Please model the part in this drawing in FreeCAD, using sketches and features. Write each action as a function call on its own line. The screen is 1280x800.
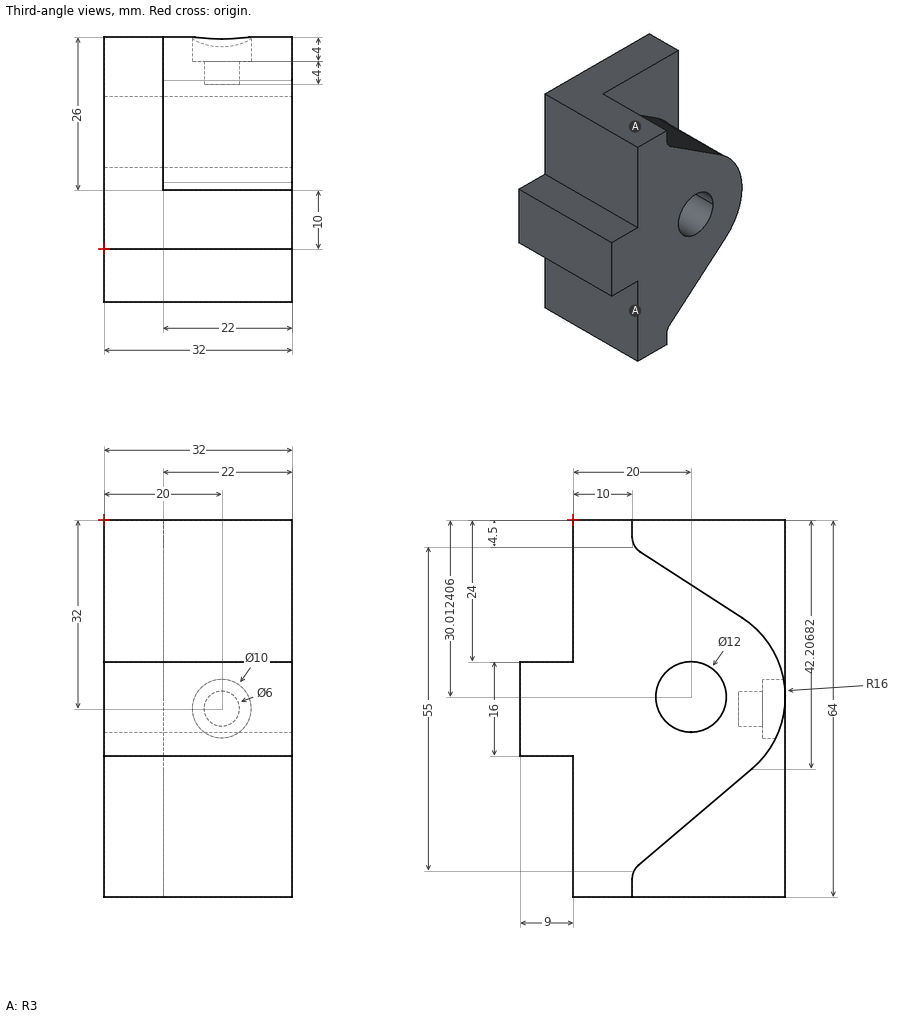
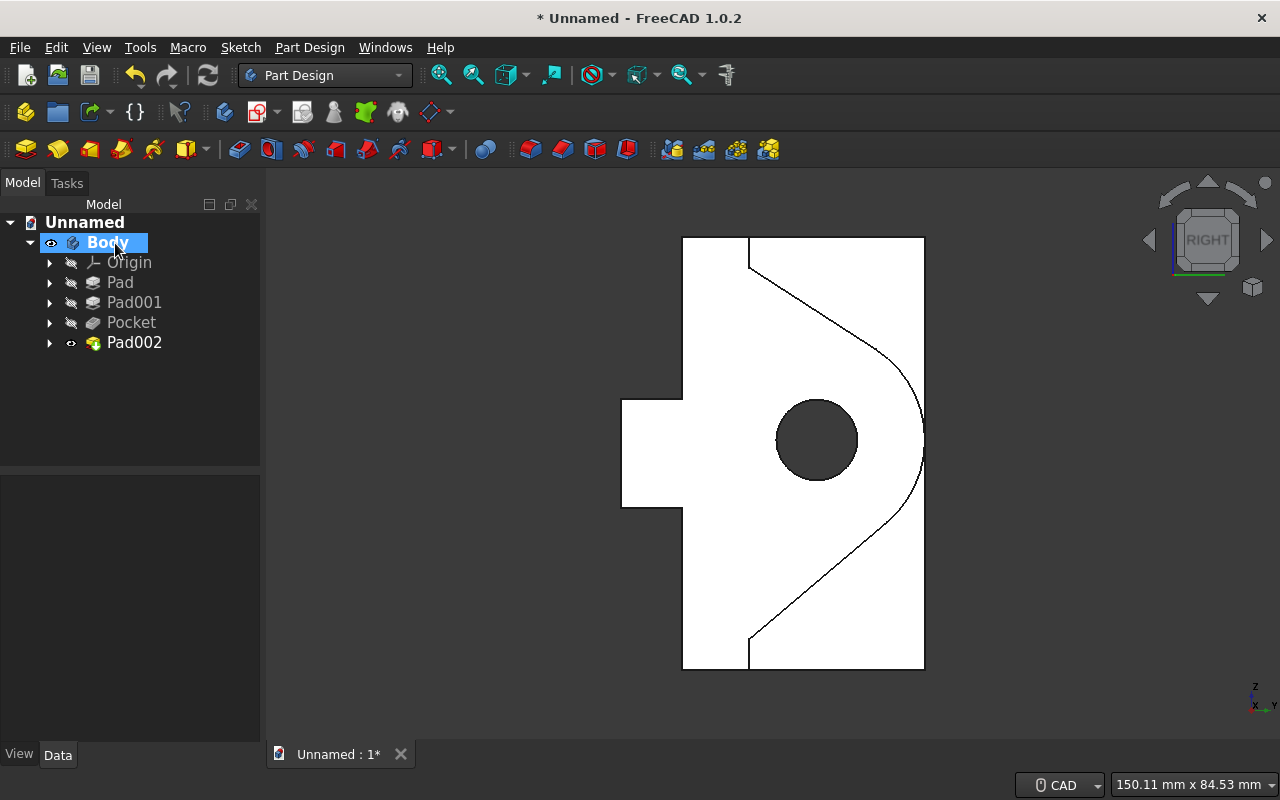
key(5)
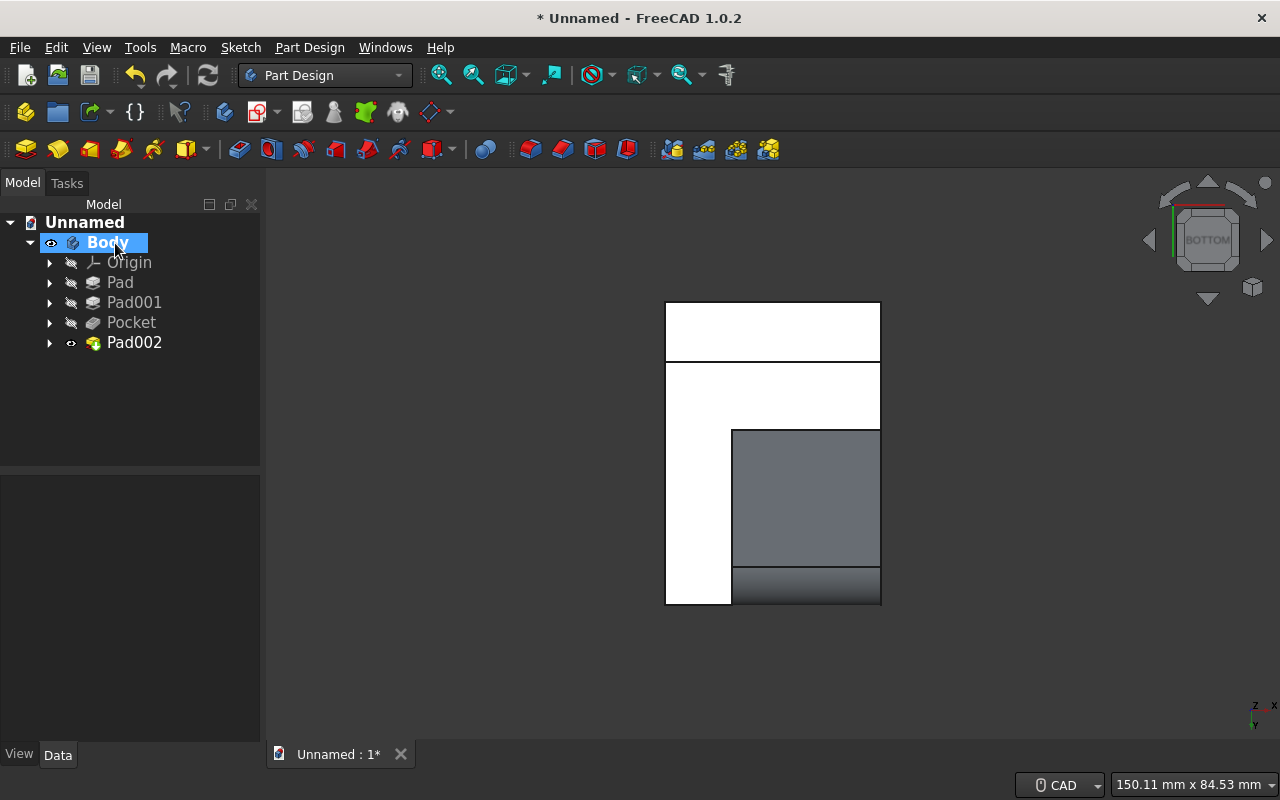
key(4)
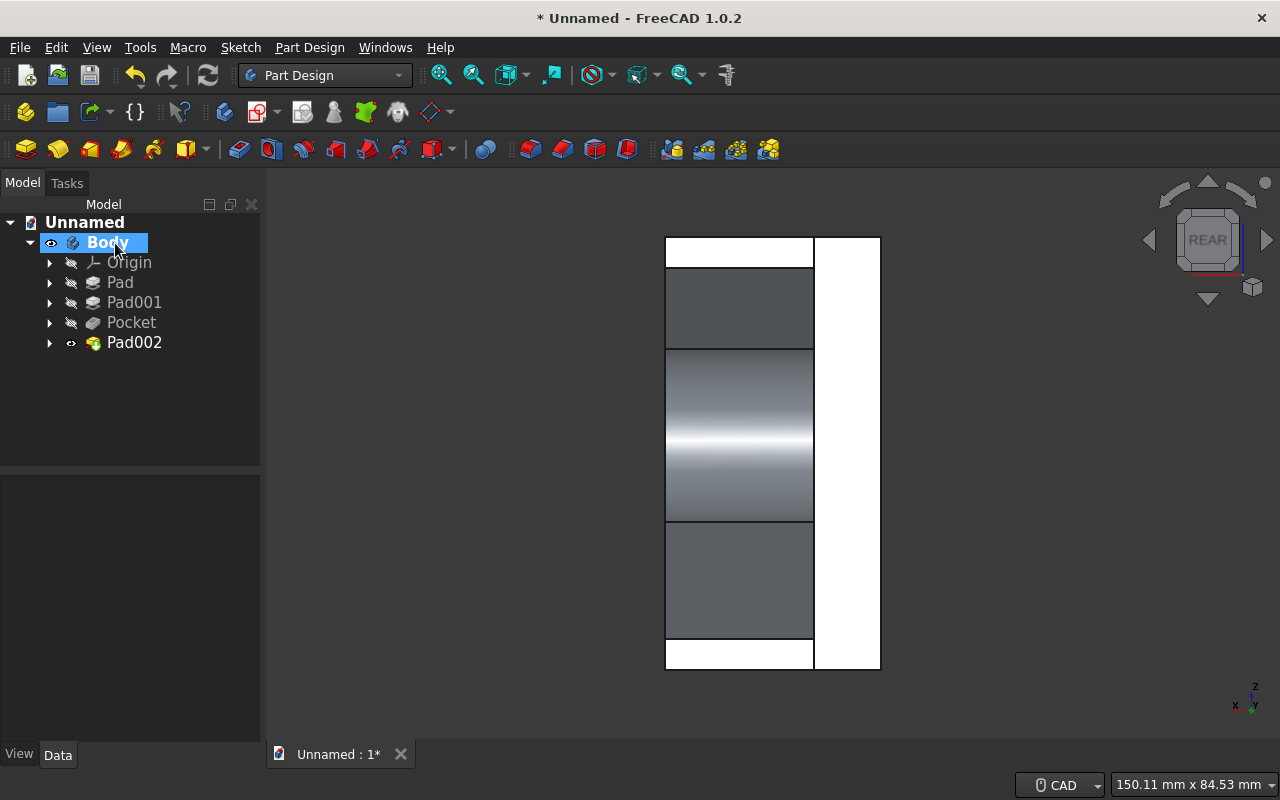
key(6)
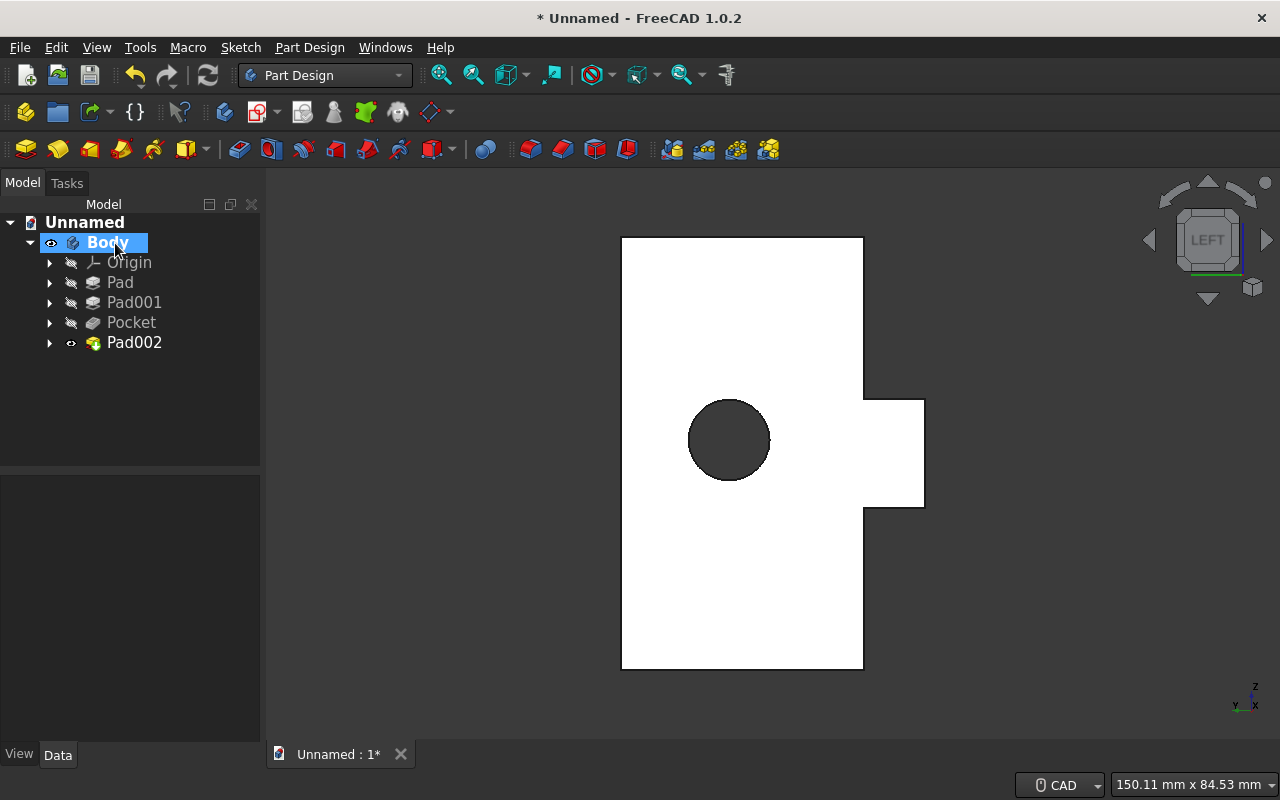
key(v)
key(3)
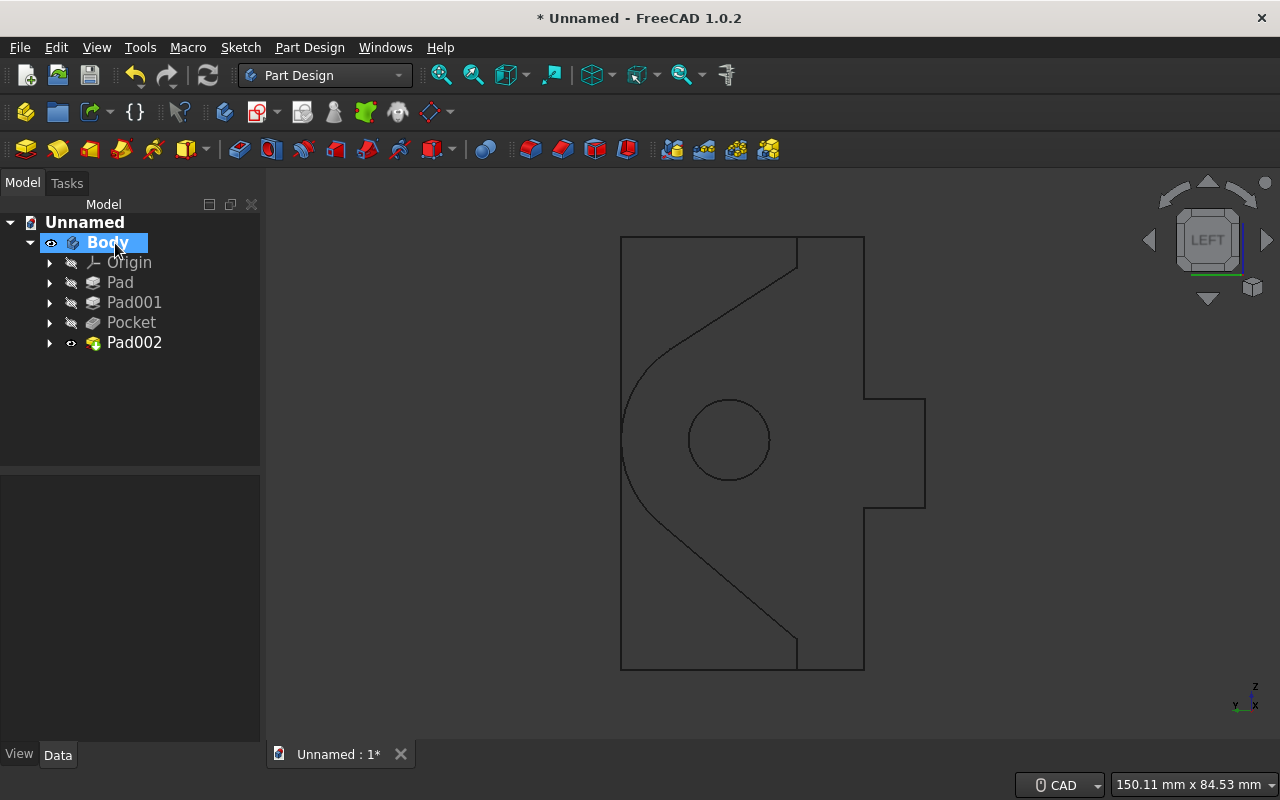
key(0)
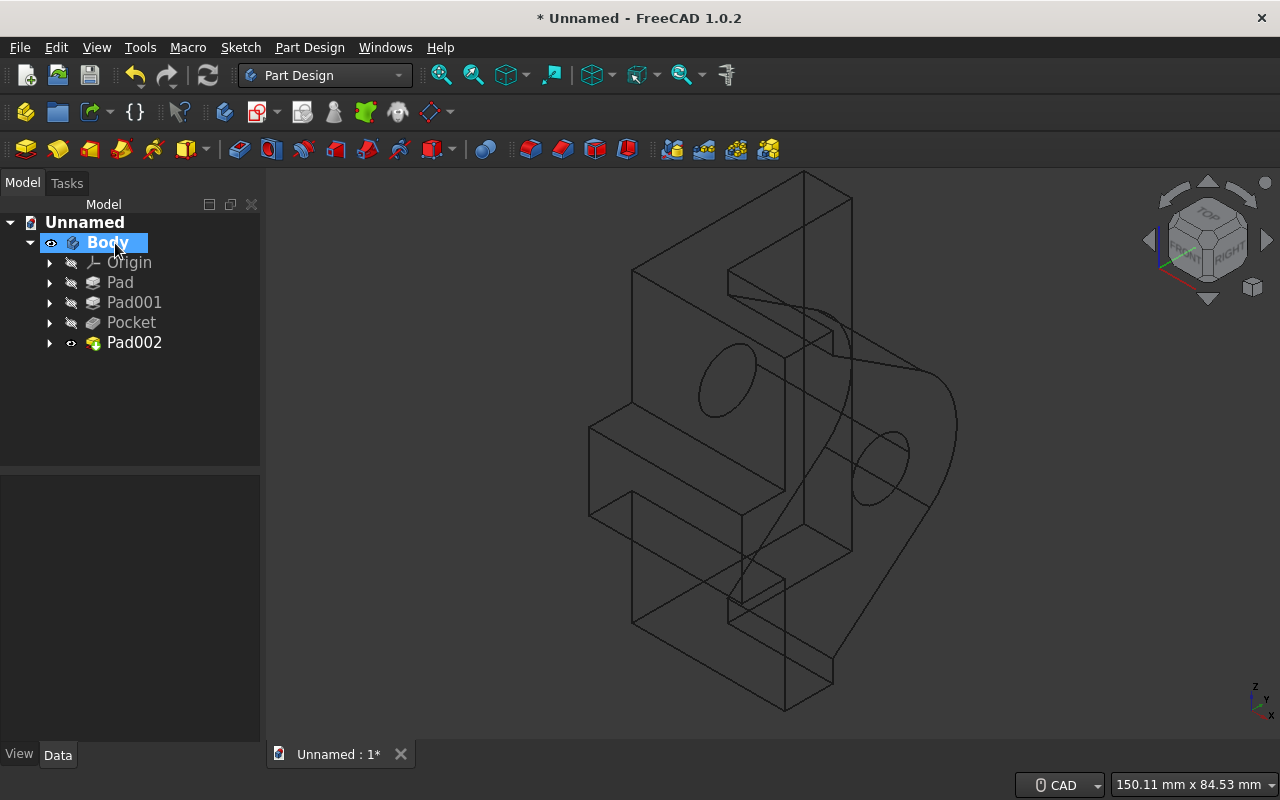
click(791, 634)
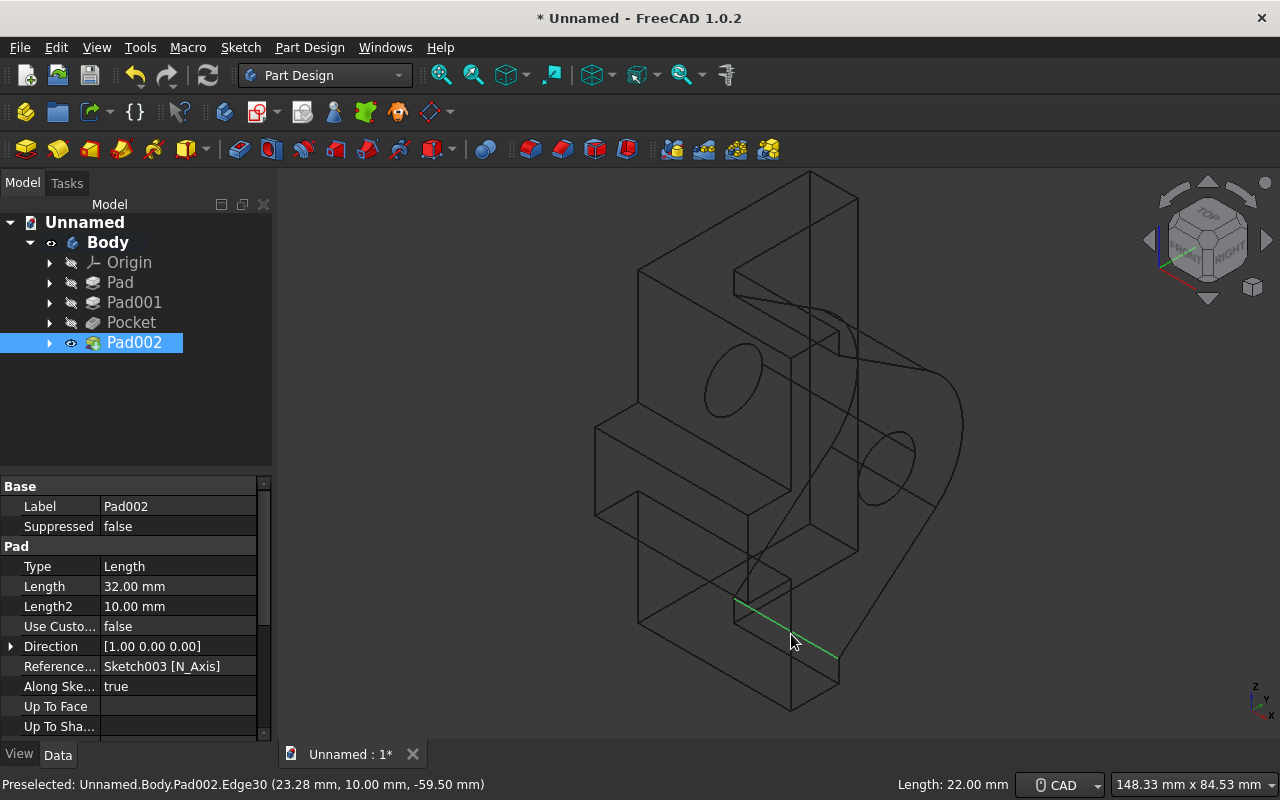
click(786, 324, ctrl)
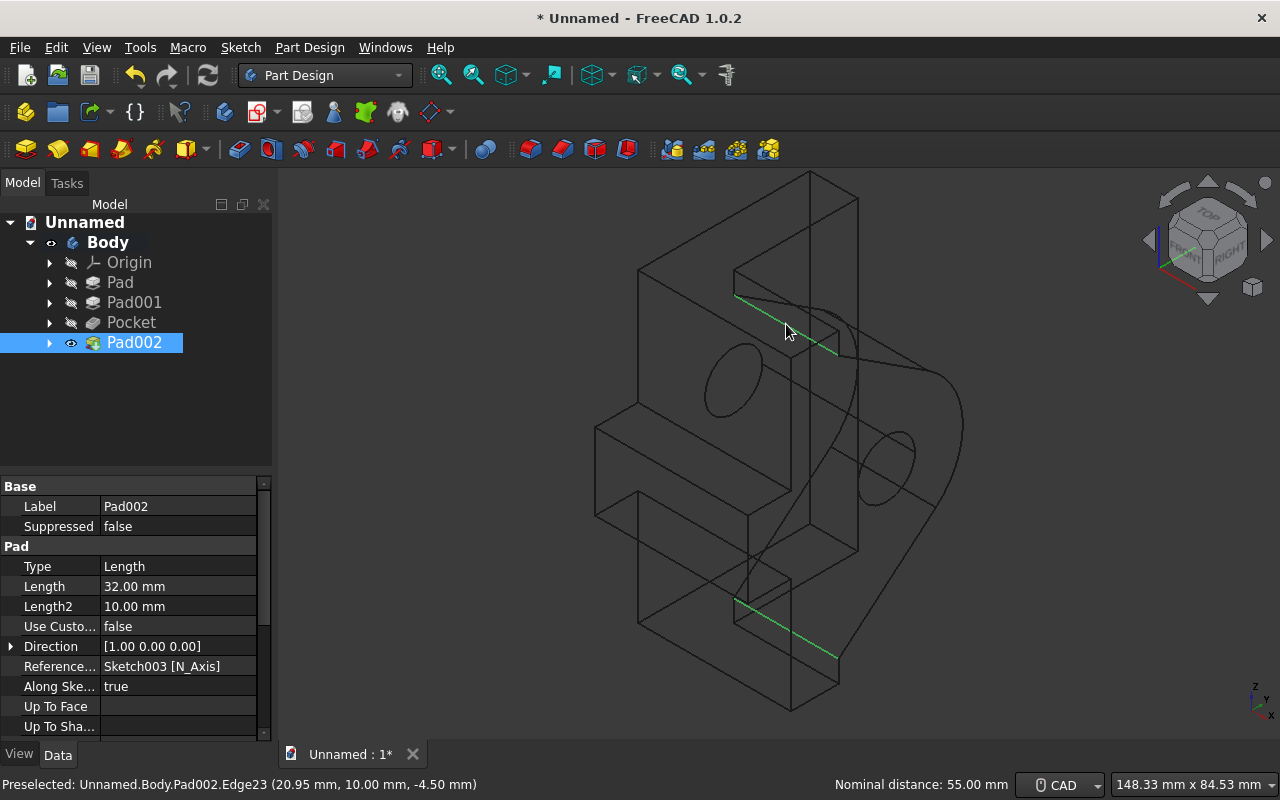
key(v)
key(1)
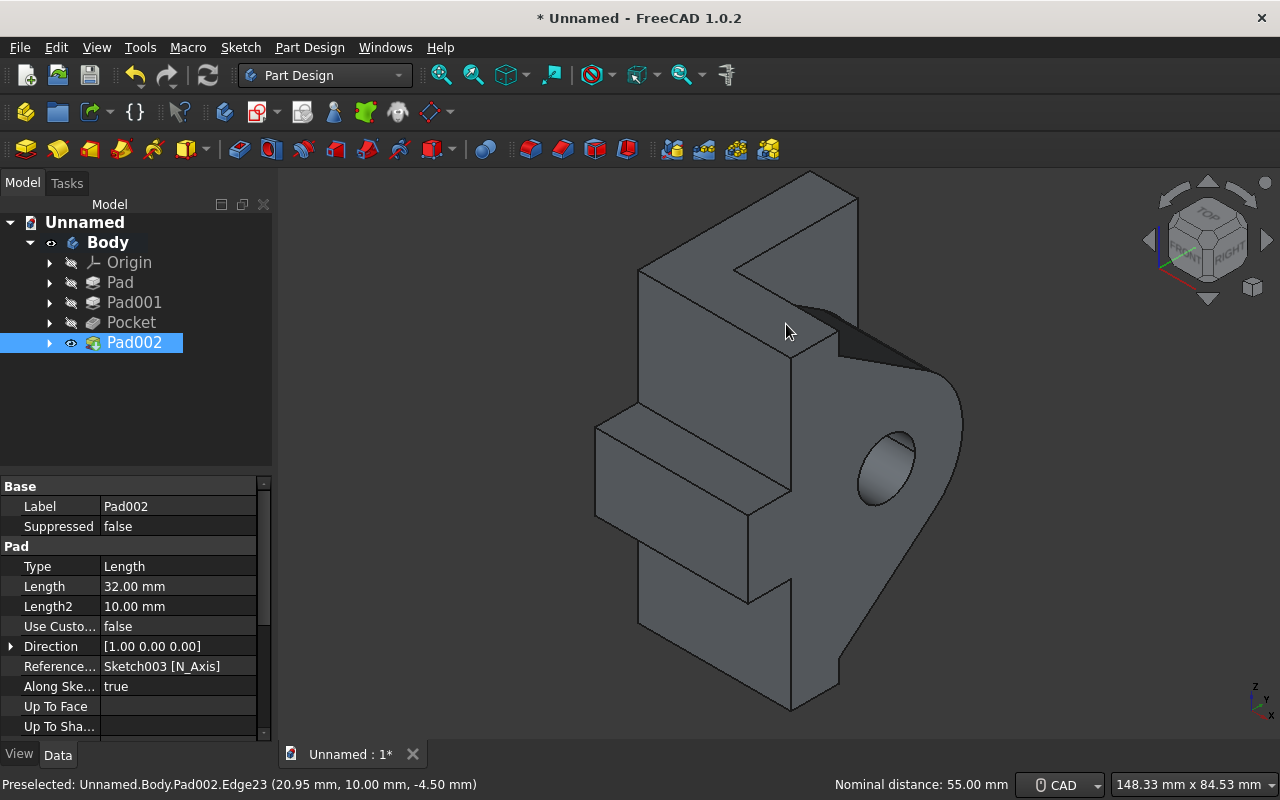
click(532, 150)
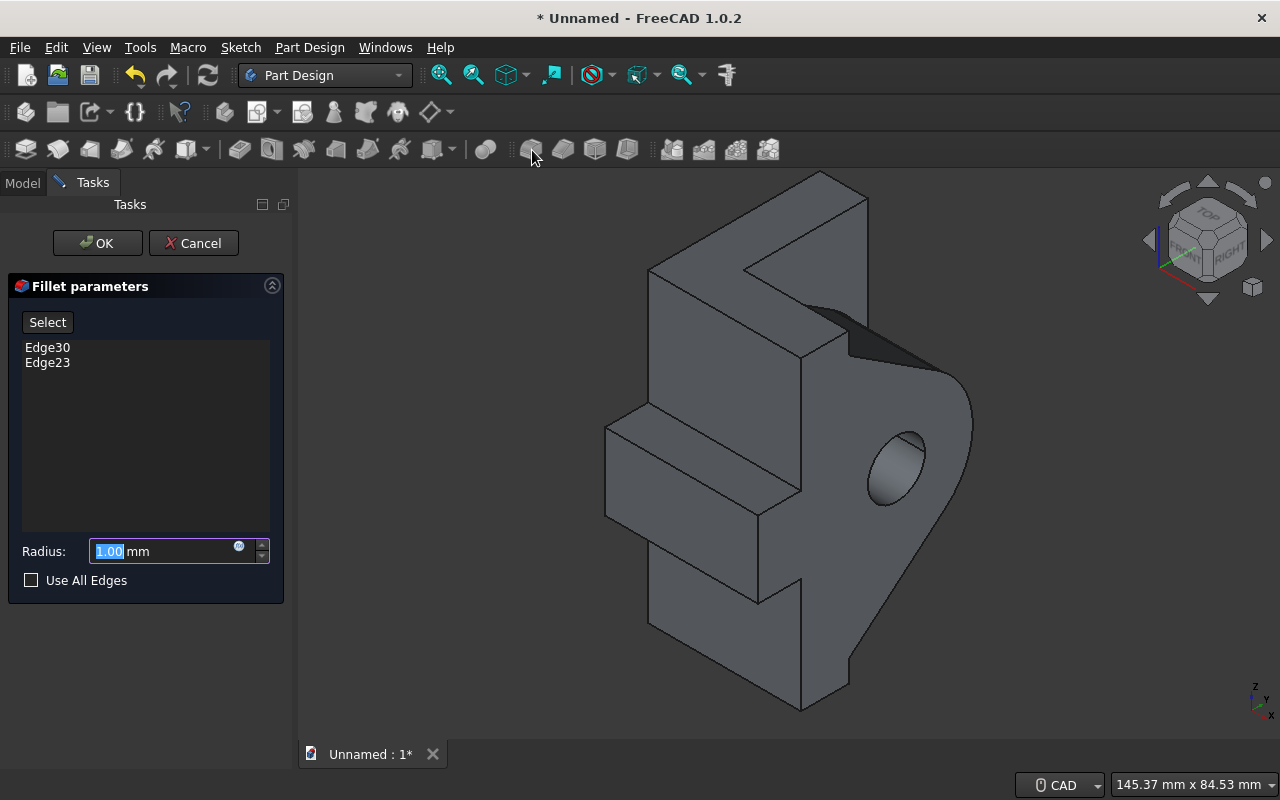
text(3)
key(Tab)